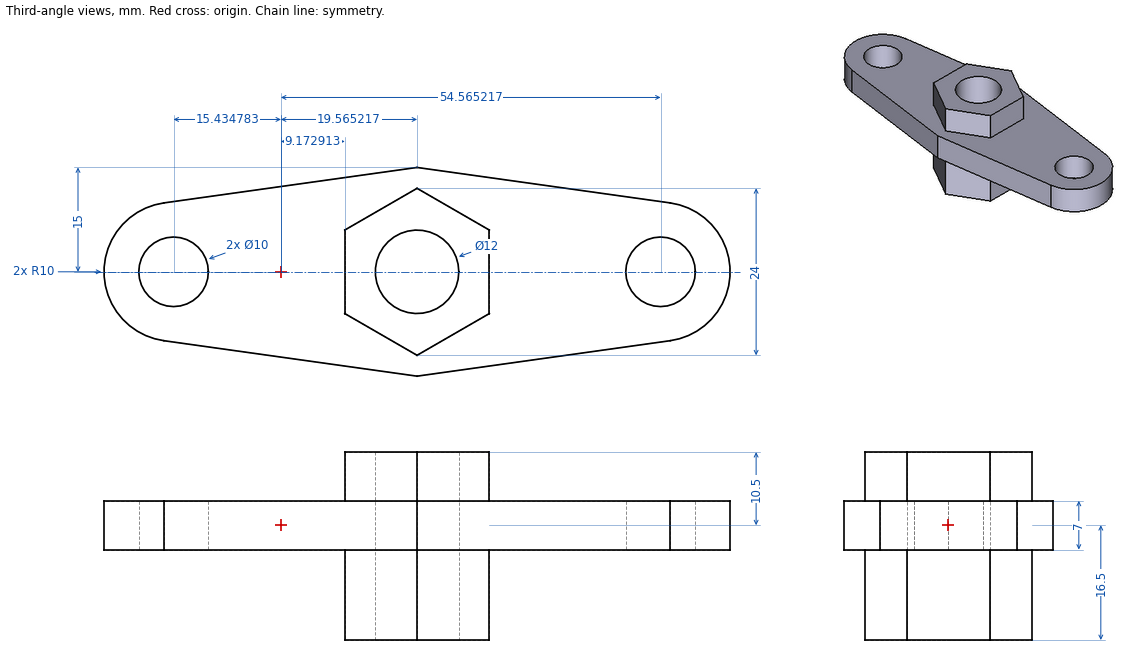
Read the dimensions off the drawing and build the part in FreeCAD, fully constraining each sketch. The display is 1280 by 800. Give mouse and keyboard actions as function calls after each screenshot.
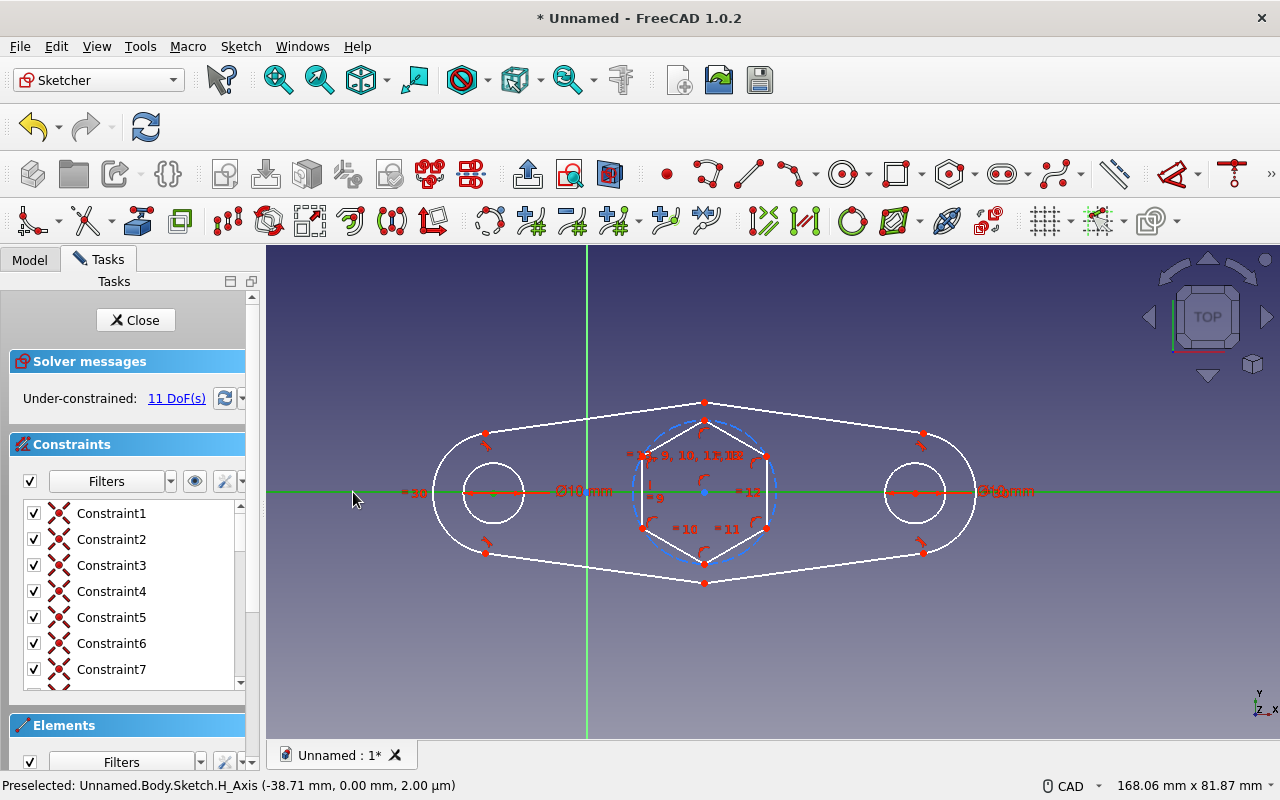
click(1232, 174)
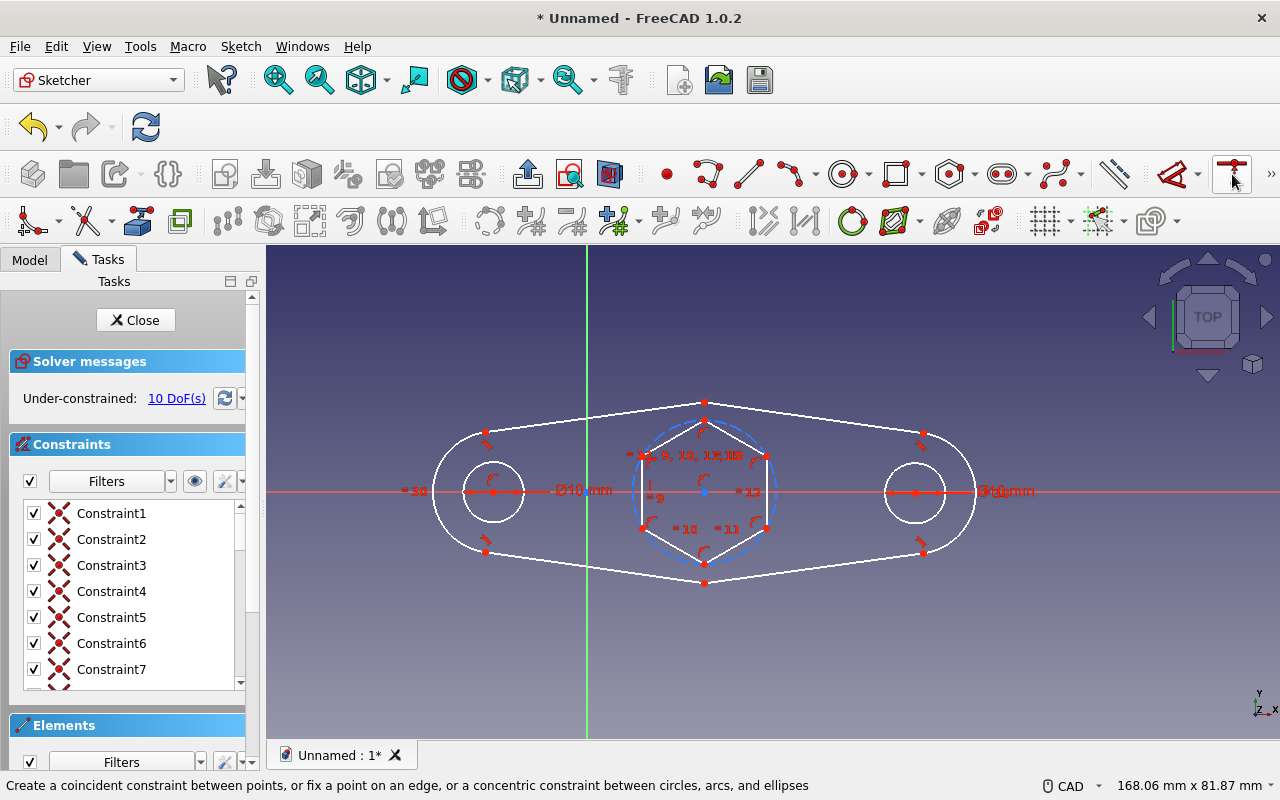
click(915, 493)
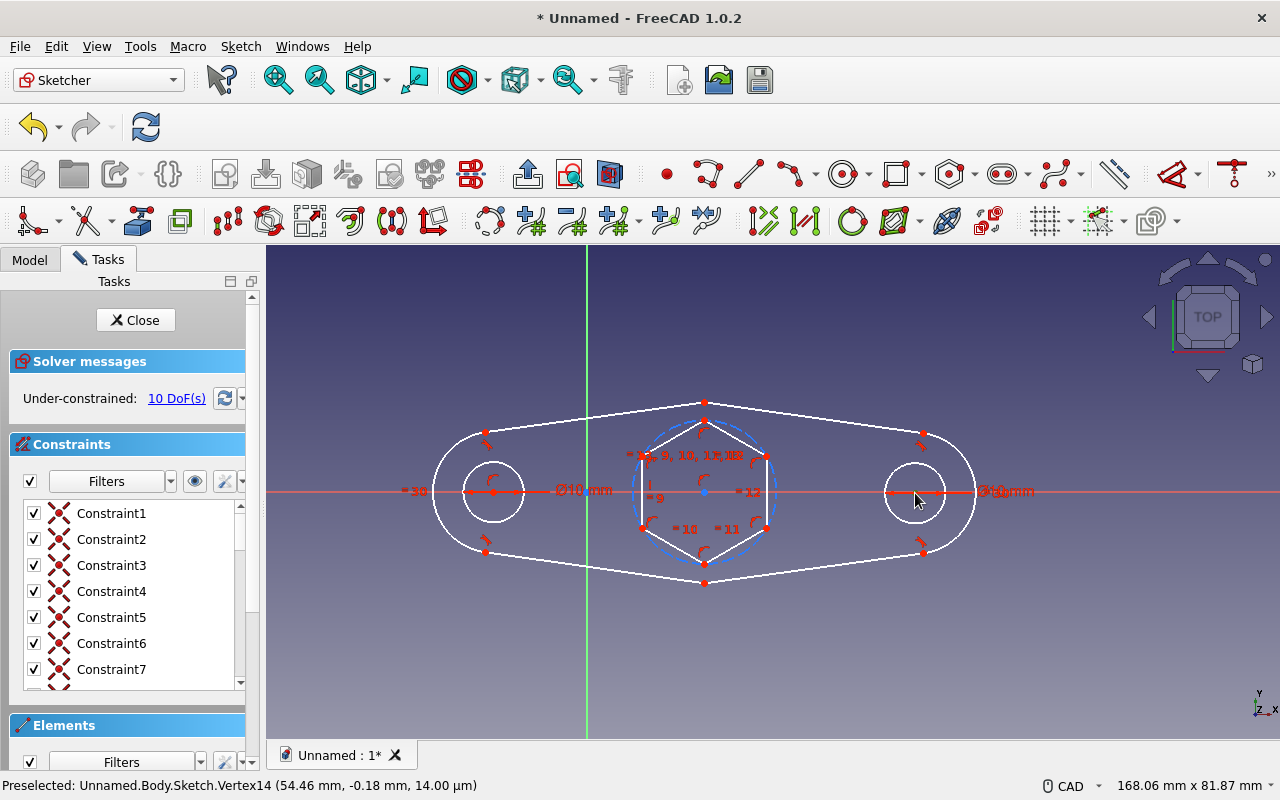
click(353, 492)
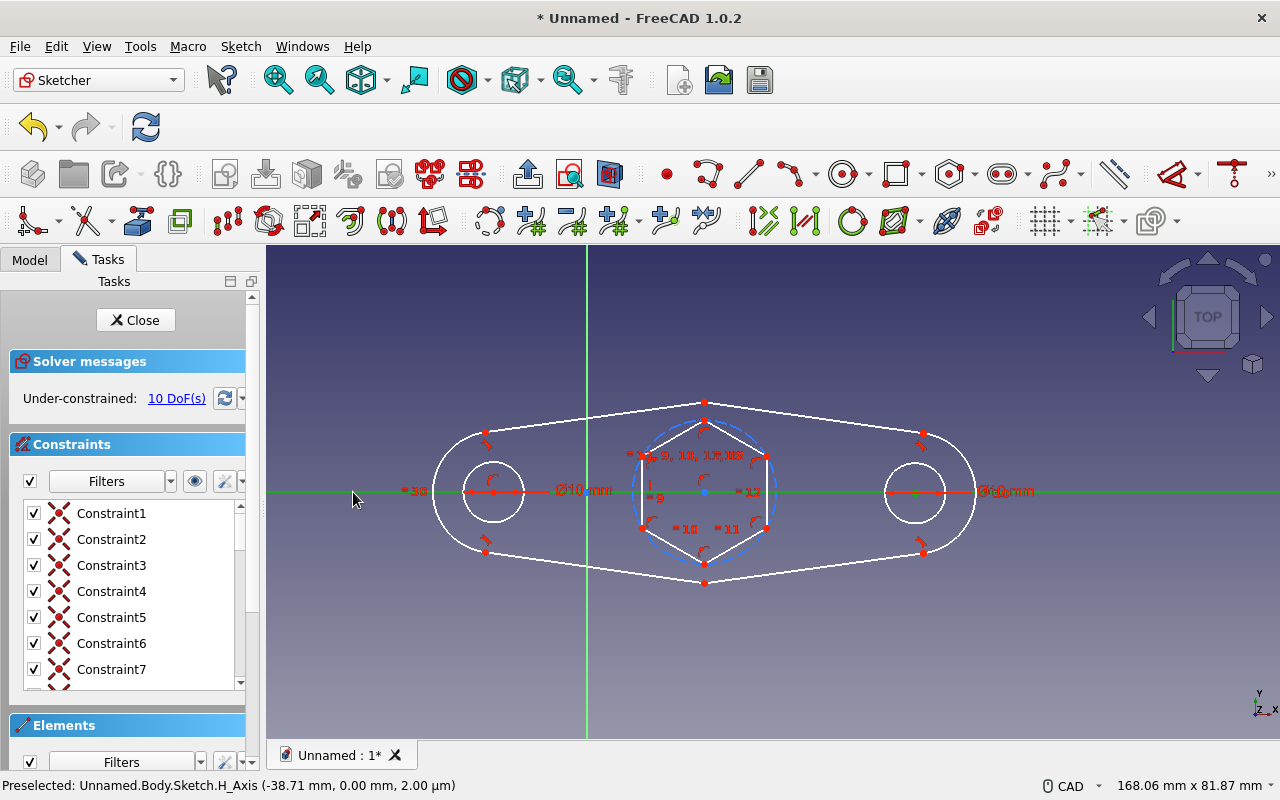
click(1232, 174)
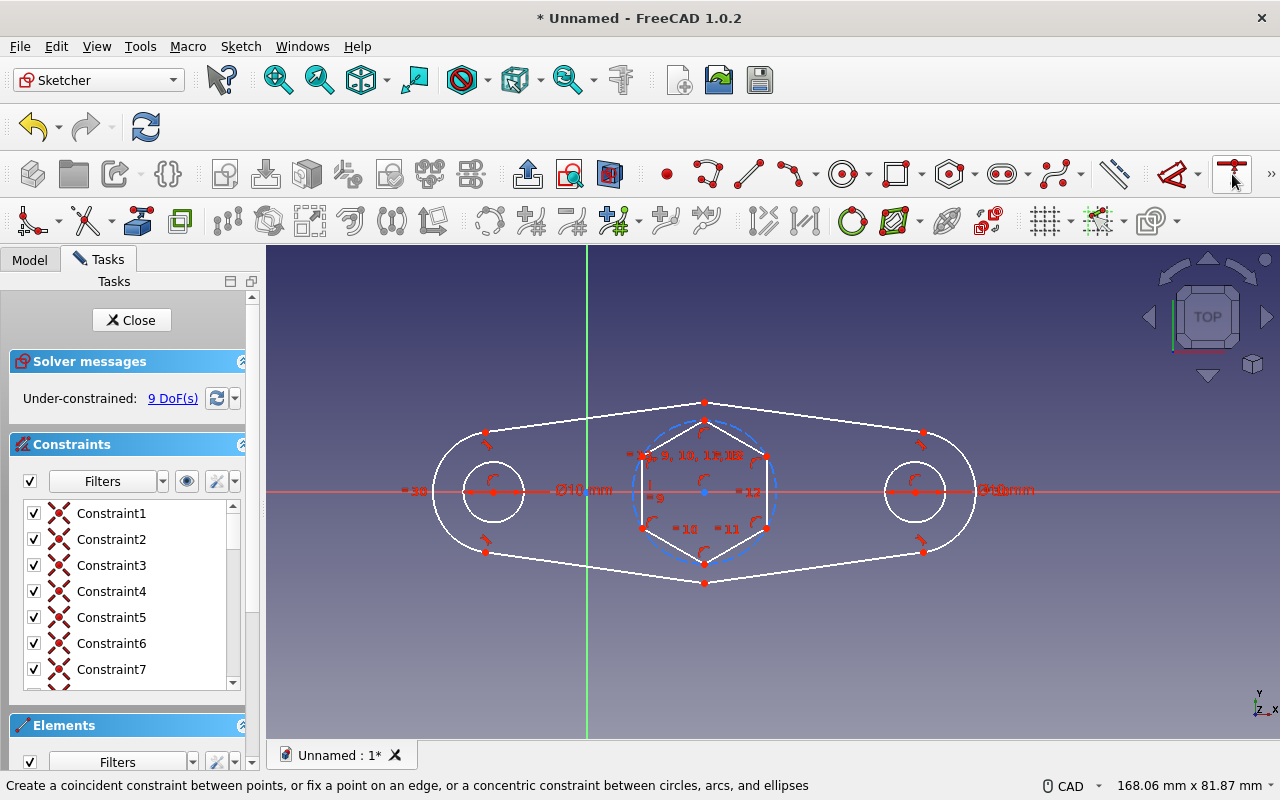
click(704, 402)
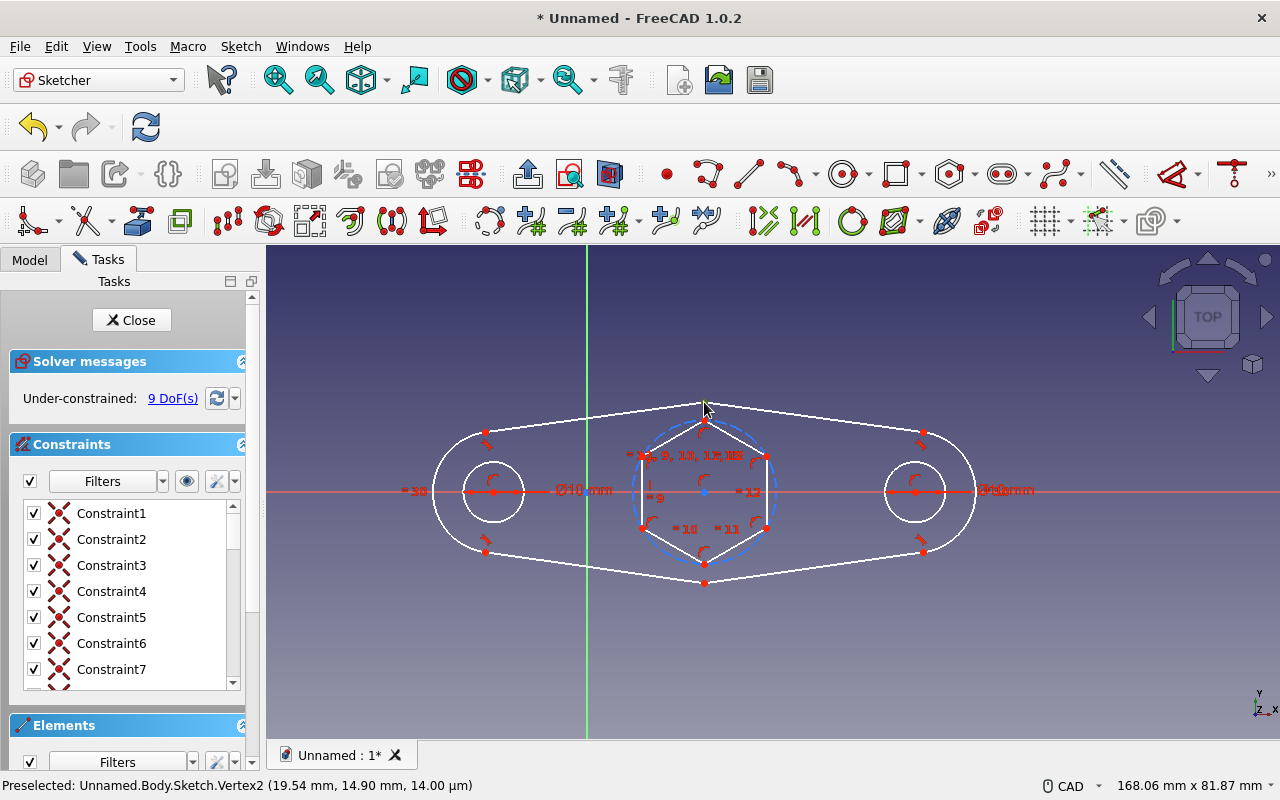
click(704, 583)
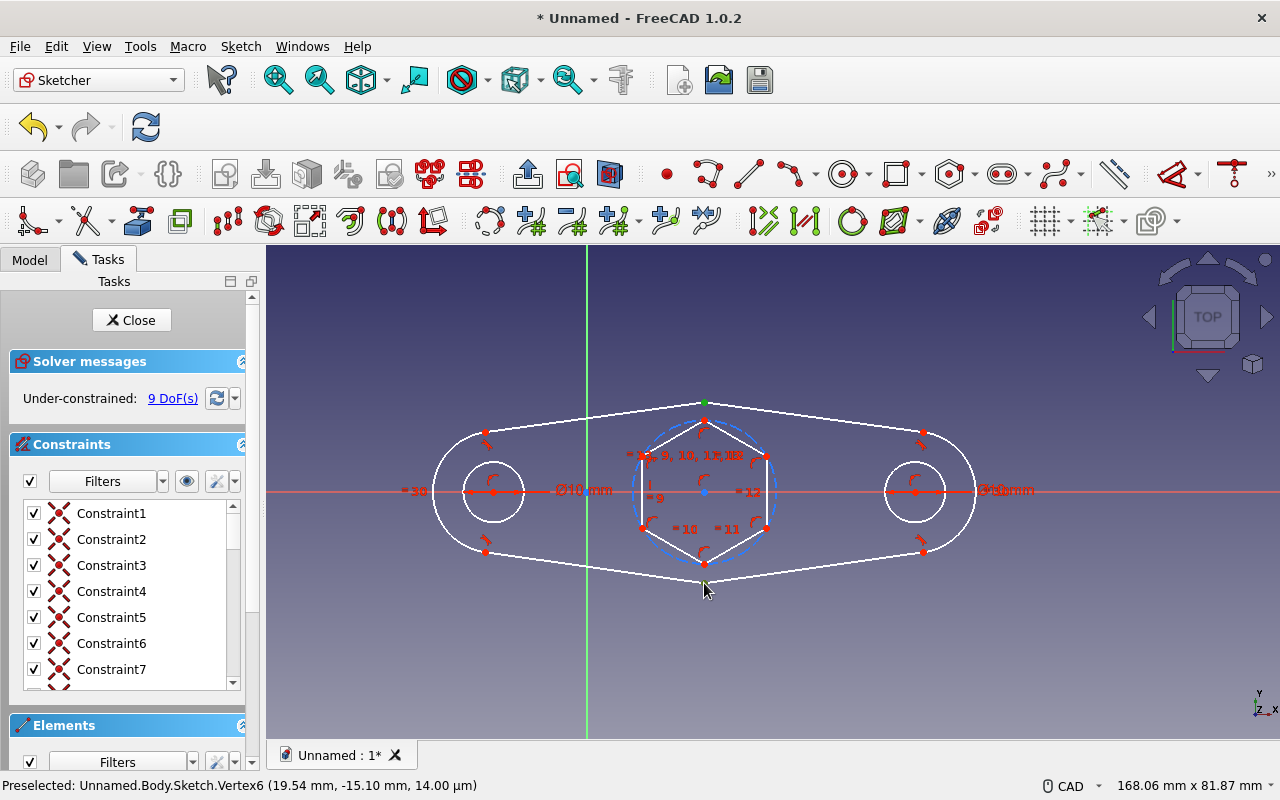
click(353, 492)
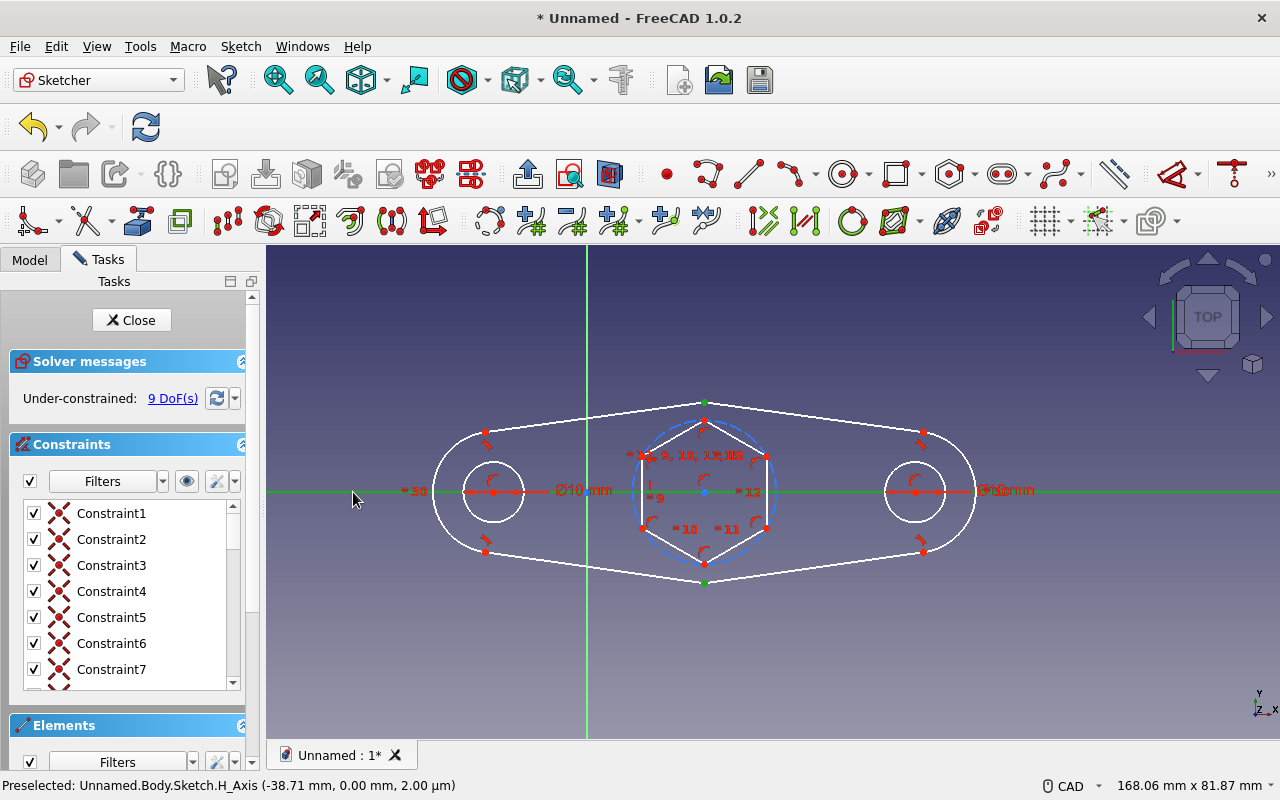
key(s)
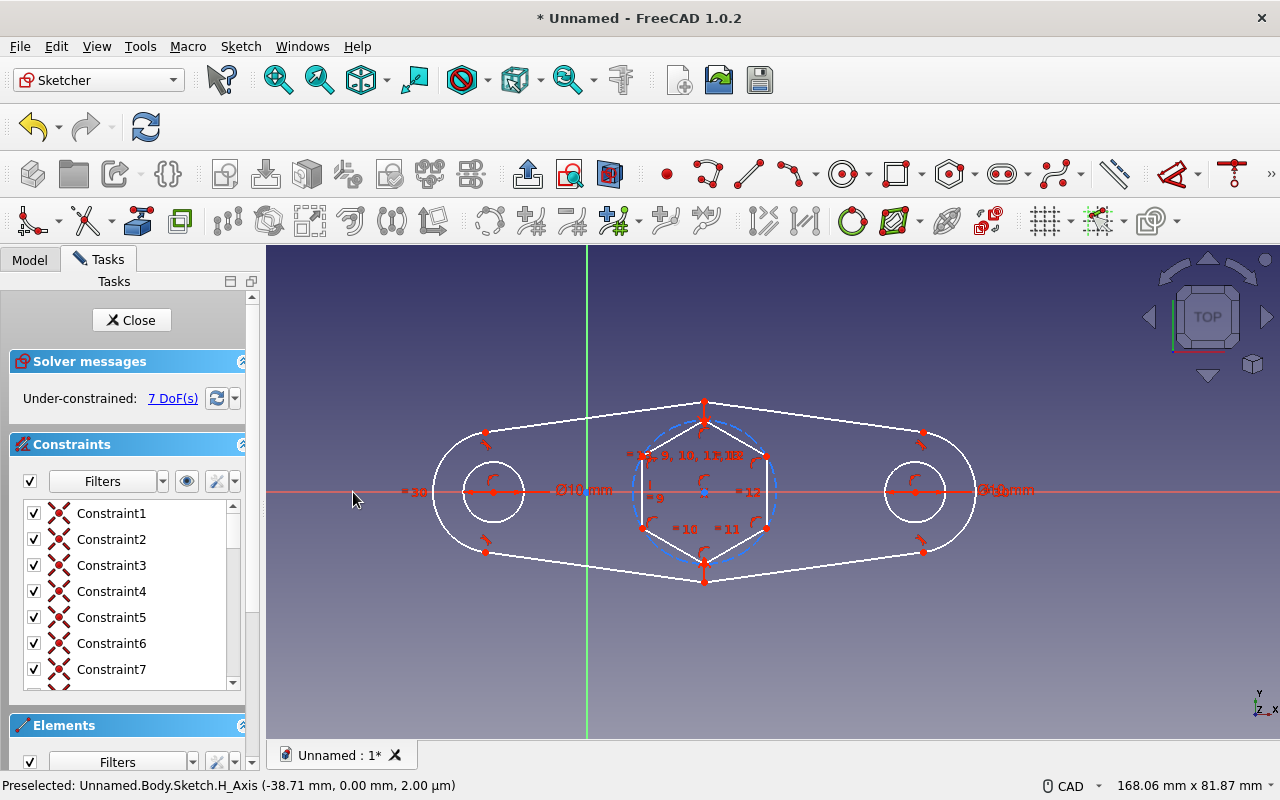
click(1172, 174)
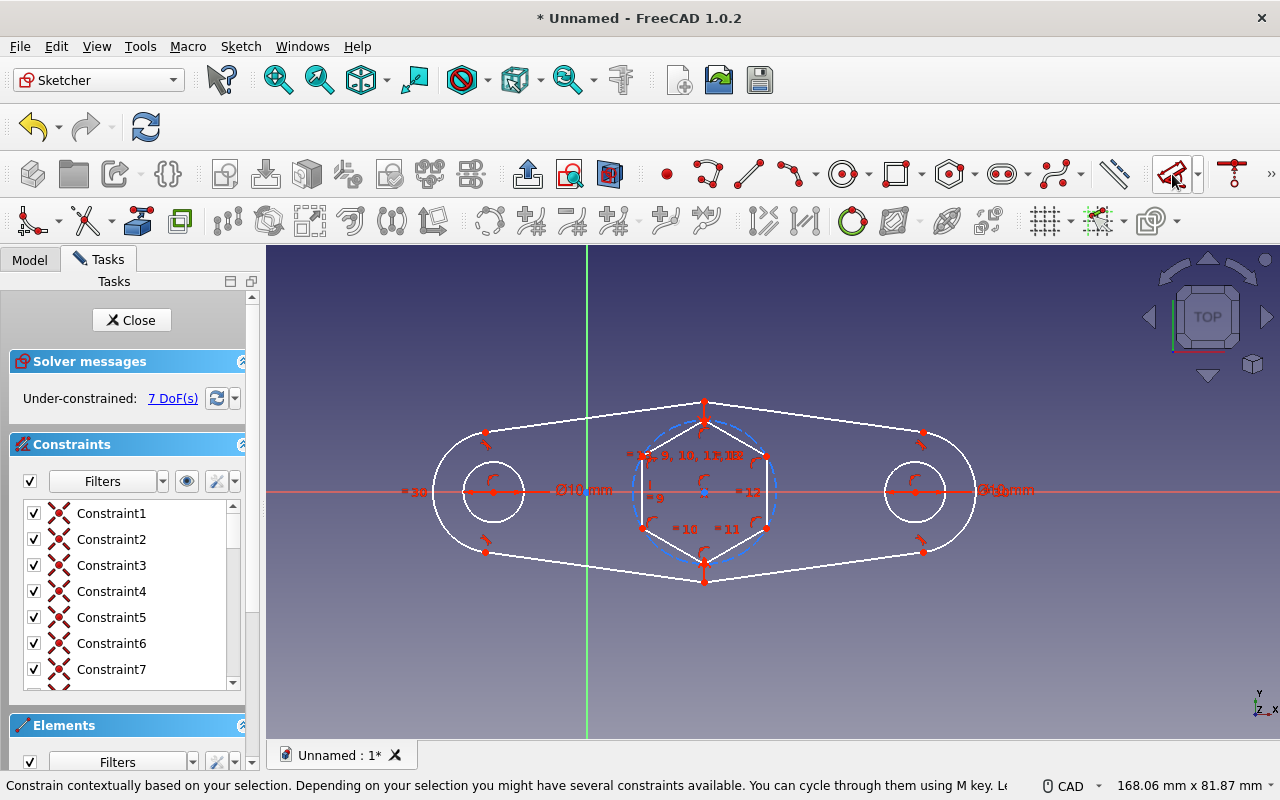
click(443, 459)
click(416, 441)